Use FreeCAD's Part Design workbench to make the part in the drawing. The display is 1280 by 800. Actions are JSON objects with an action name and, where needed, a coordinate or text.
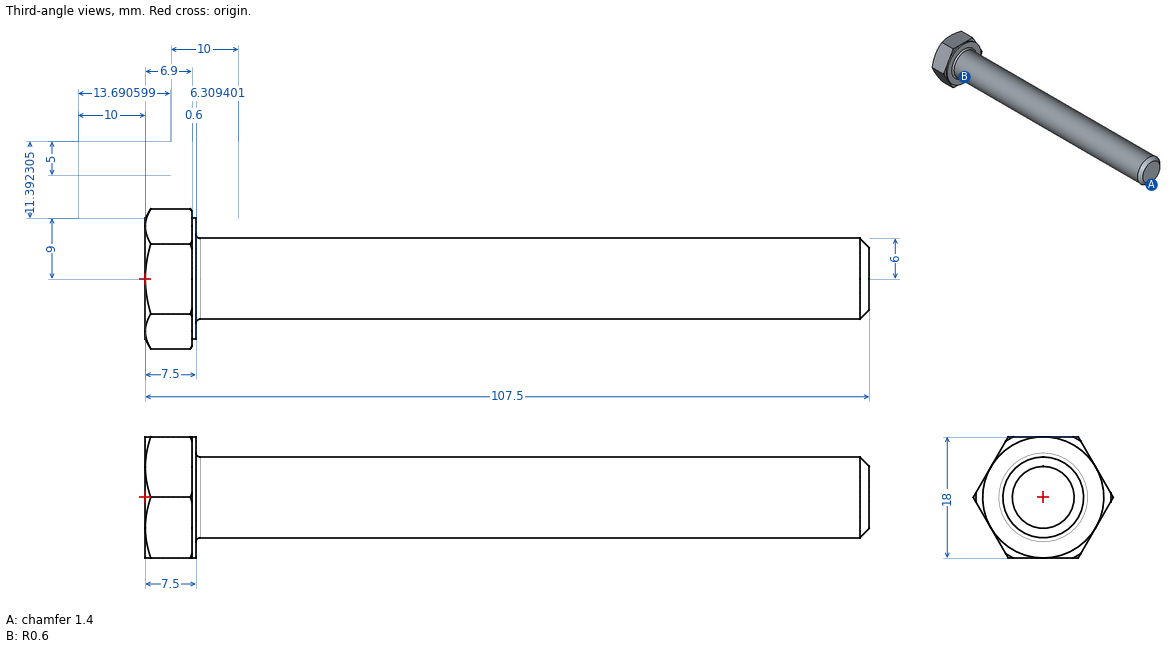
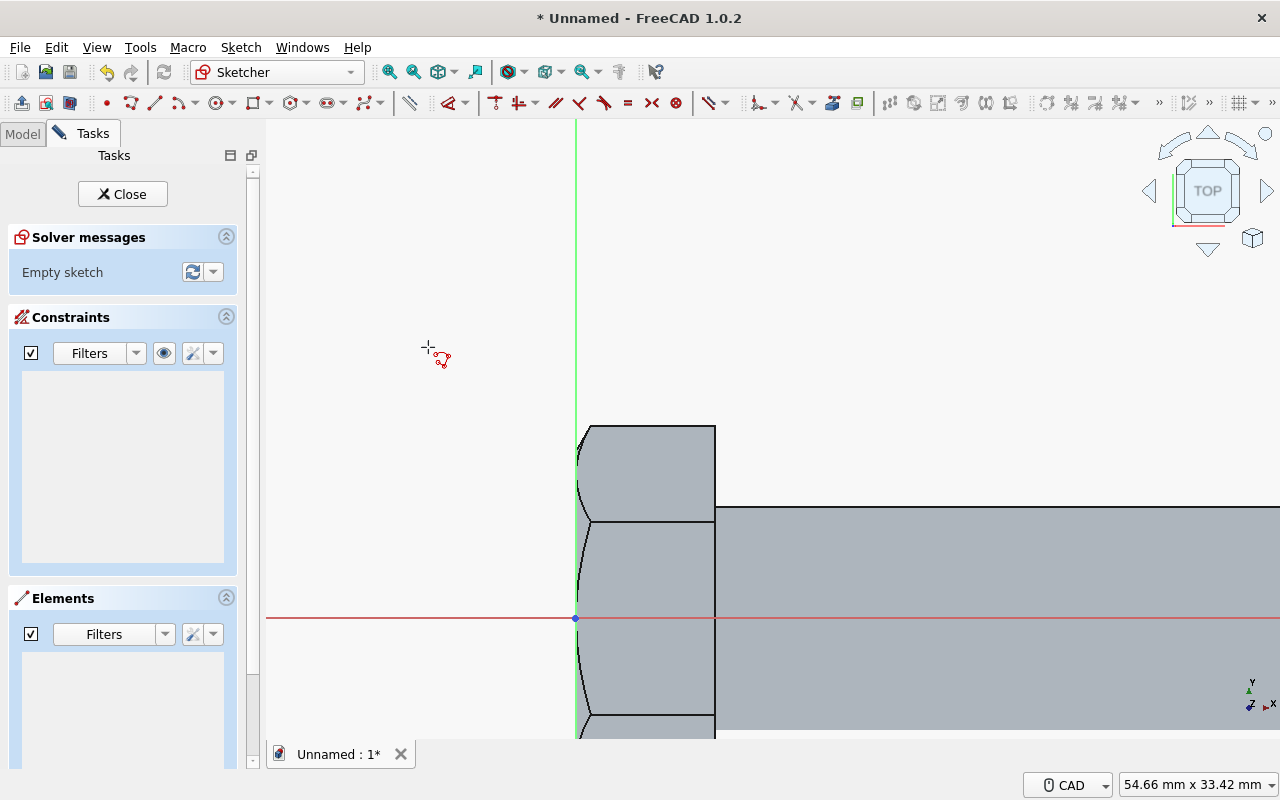
{"action": "left_click", "coordinate": [715, 451]}
{"action": "left_click", "coordinate": [832, 451]}
{"action": "left_click", "coordinate": [832, 240]}
{"action": "left_click", "coordinate": [647, 240]}
{"action": "left_click", "coordinate": [647, 333]}
{"action": "left_click", "coordinate": [715, 452]}
{"action": "key", "text": "Escape"}
{"action": "key", "text": "Escape"}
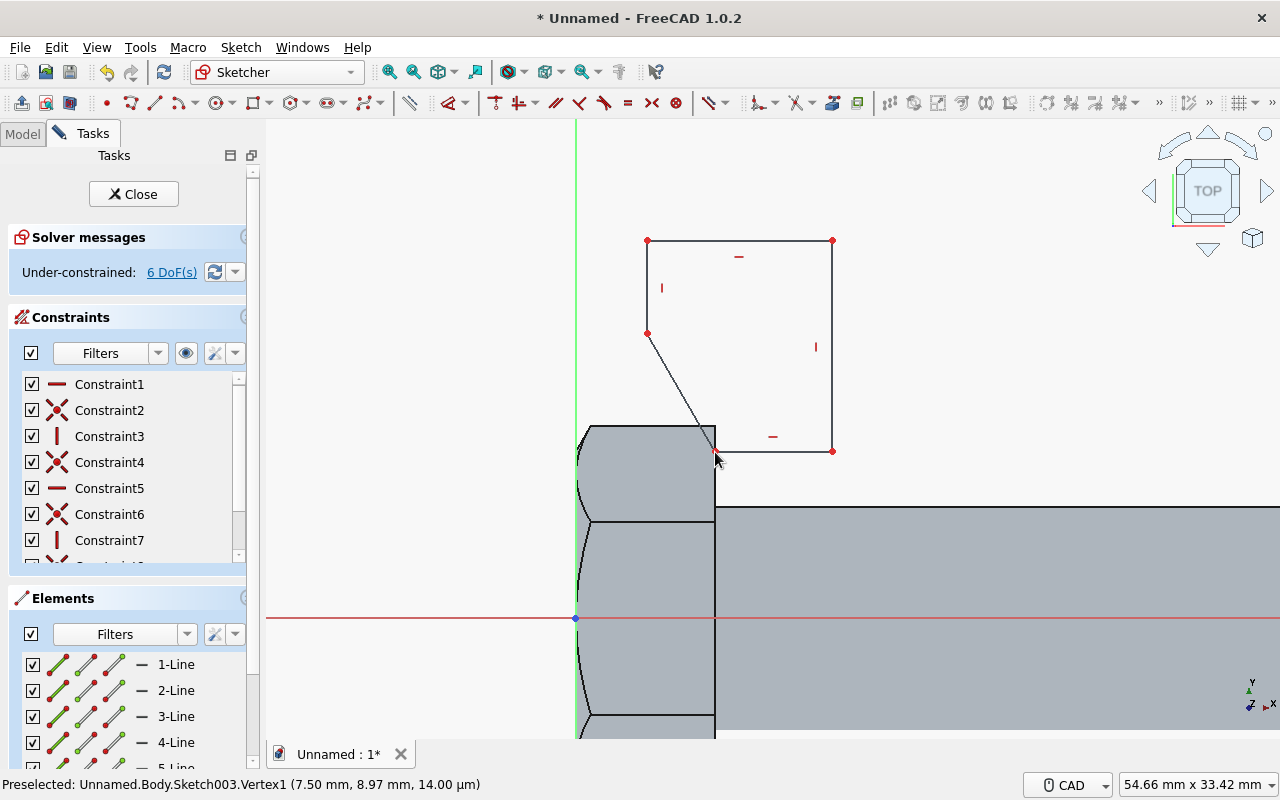
{"action": "key", "text": "d"}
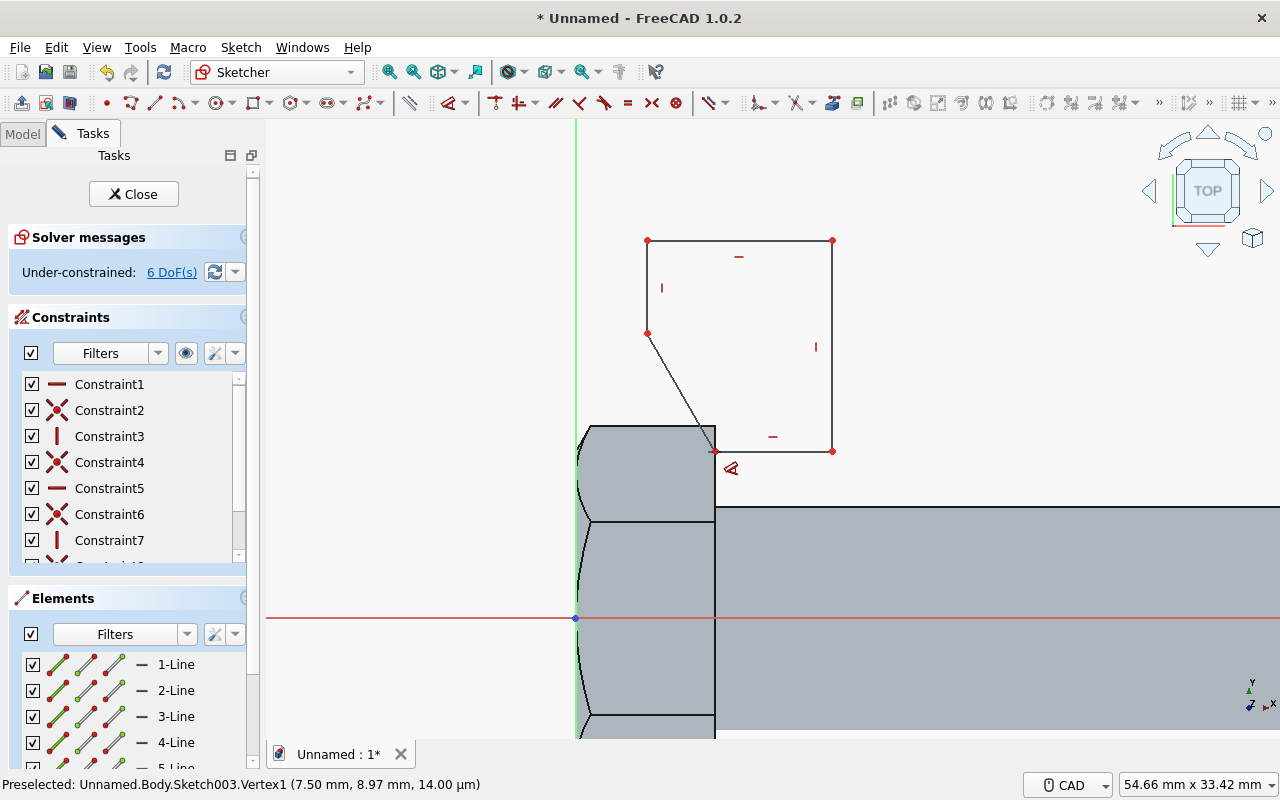
{"action": "left_click", "coordinate": [647, 269]}
{"action": "left_click", "coordinate": [613, 288]}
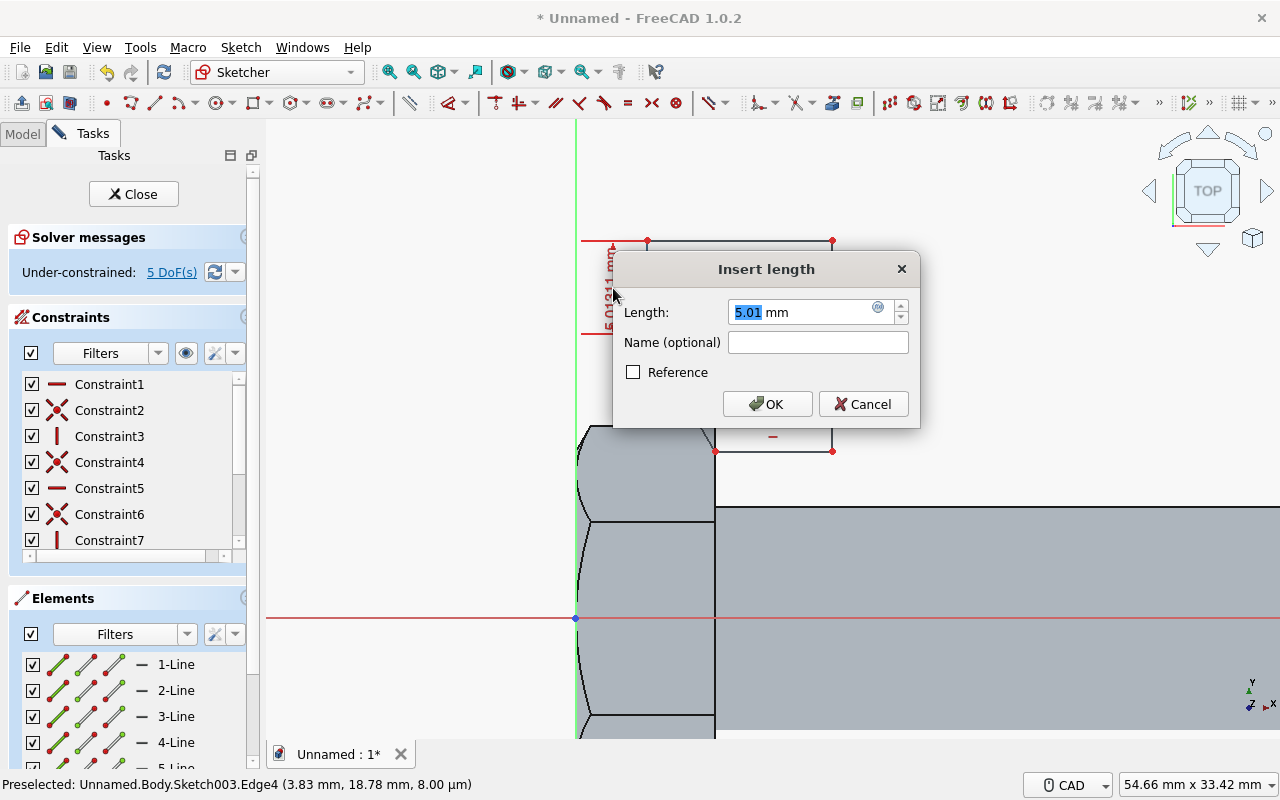
{"action": "type", "text": "5"}
{"action": "key", "text": "Return"}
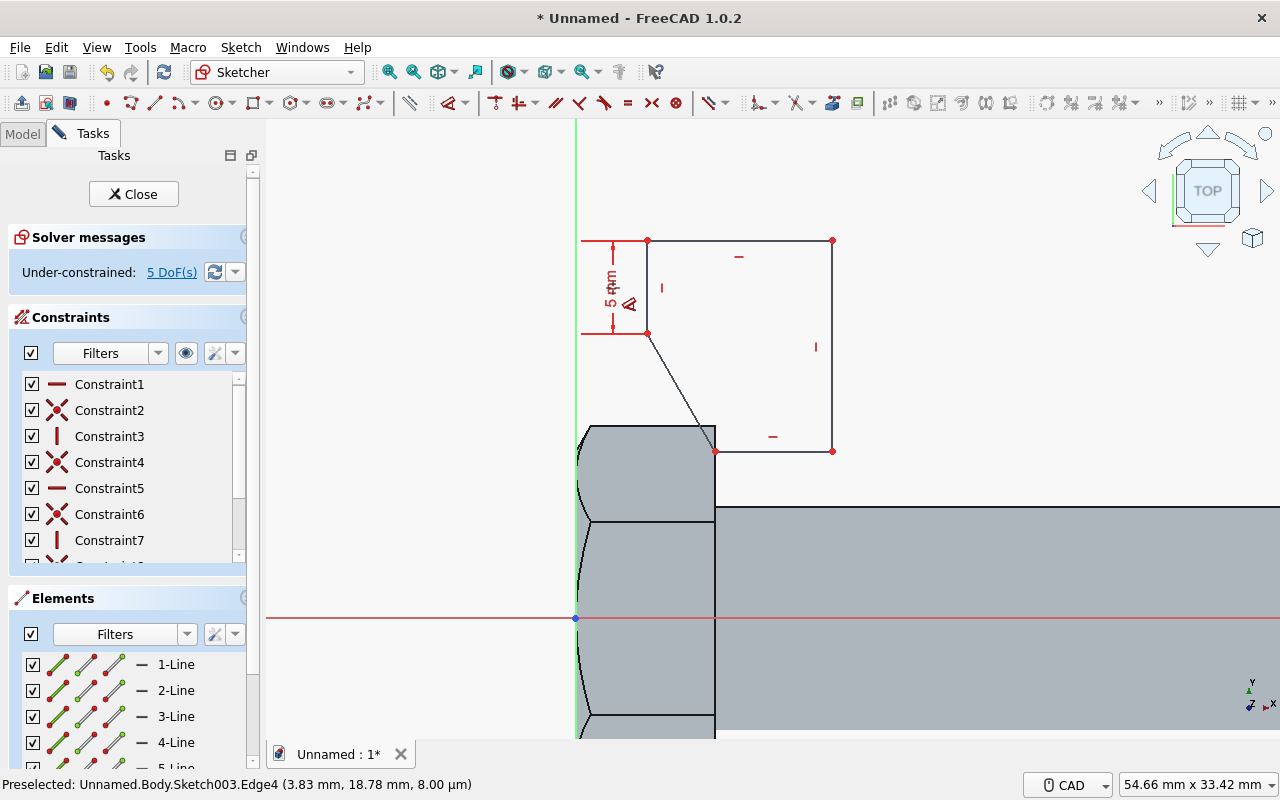
{"action": "left_click", "coordinate": [776, 241]}
{"action": "left_click", "coordinate": [739, 207]}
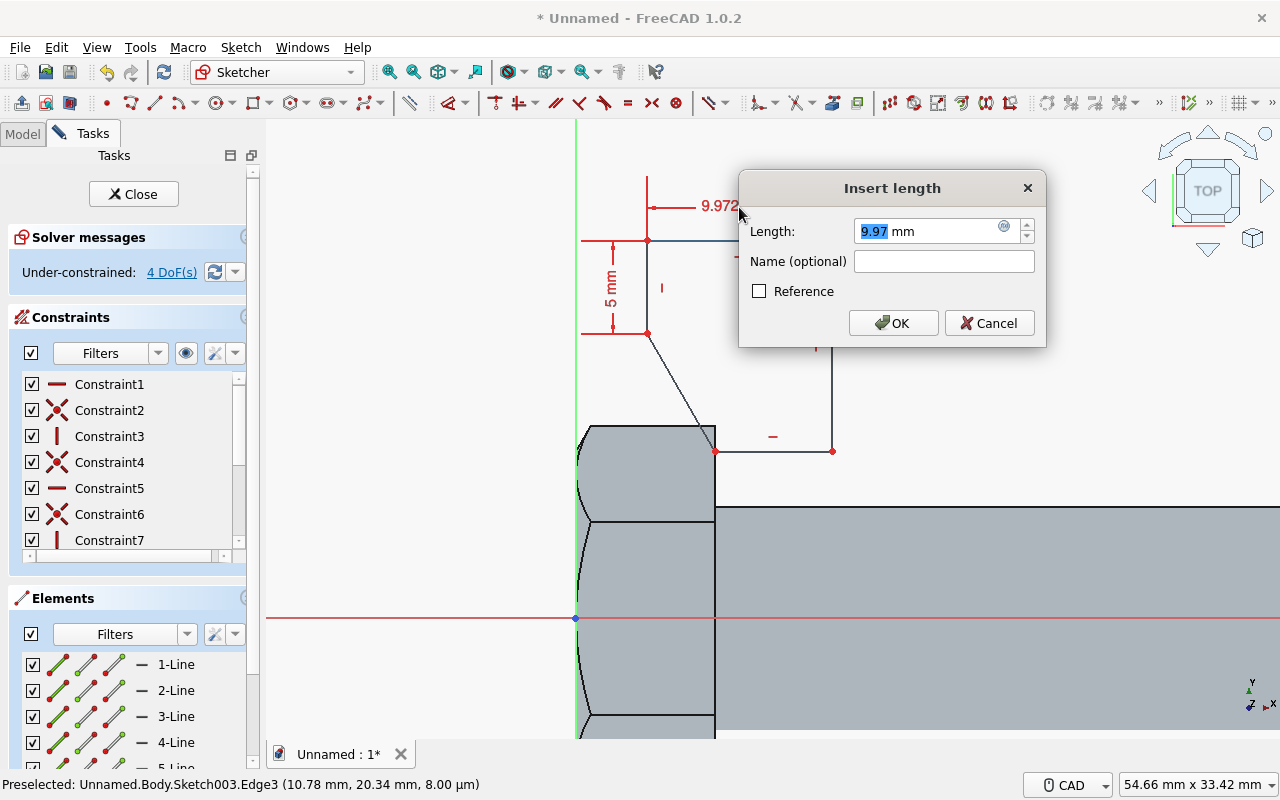
{"action": "type", "text": "10"}
{"action": "key", "text": "Return"}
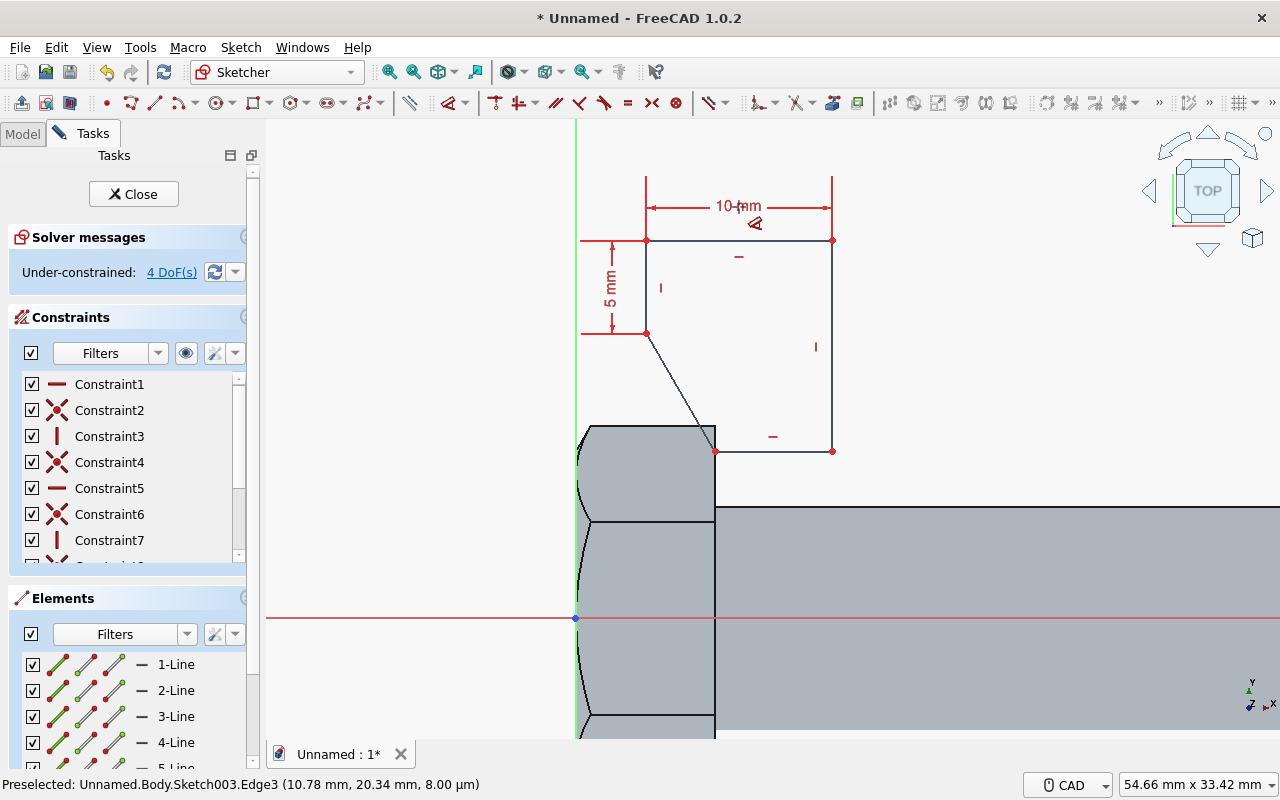
{"action": "left_click", "coordinate": [715, 452]}
{"action": "left_click", "coordinate": [542, 535]}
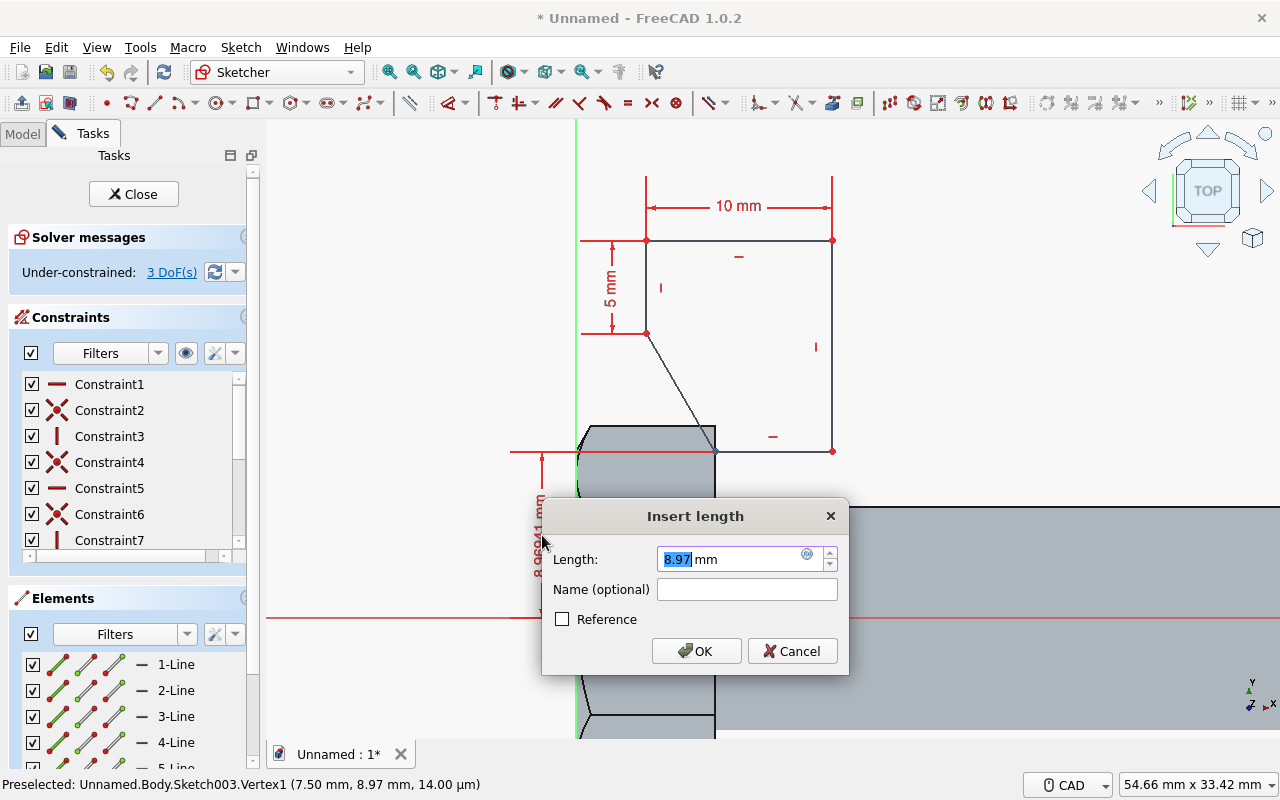
{"action": "type", "text": "9"}
{"action": "key", "text": "Return"}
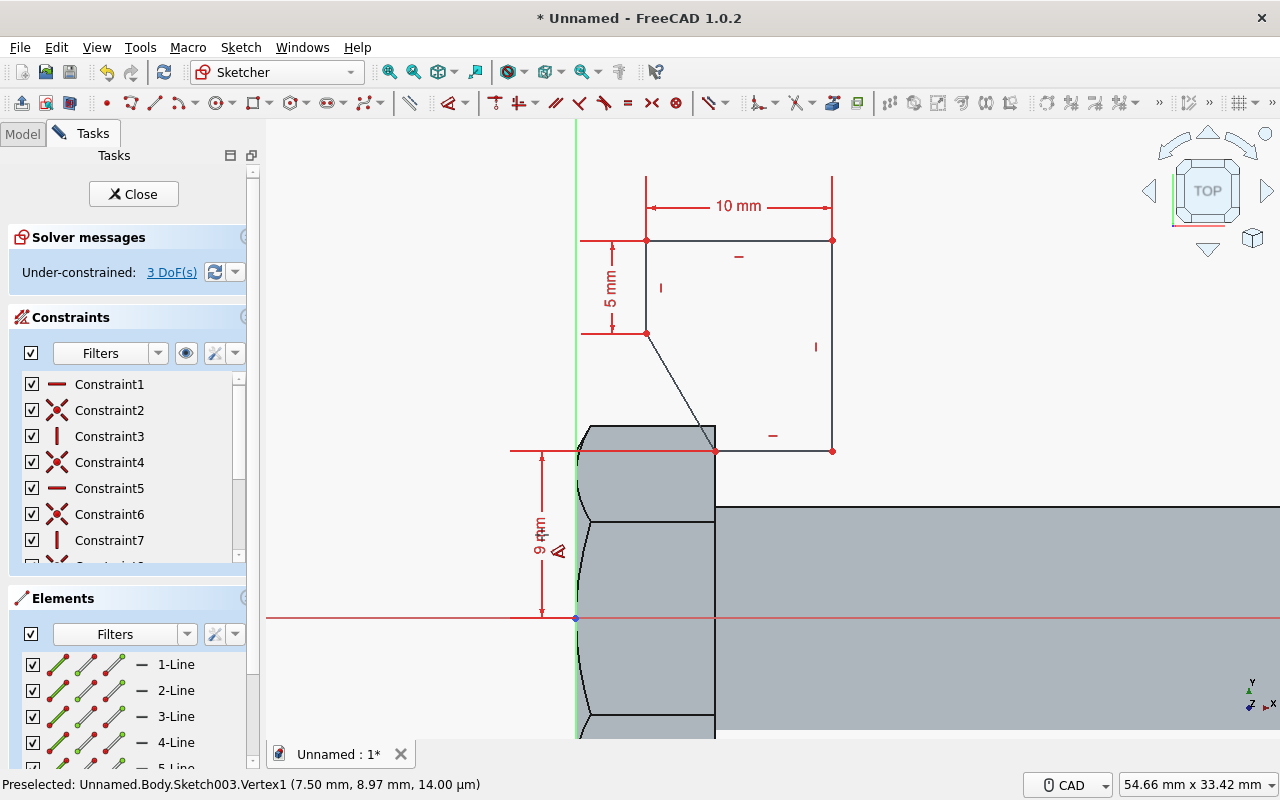
{"action": "left_click", "coordinate": [715, 451]}
{"action": "left_click", "coordinate": [645, 652]}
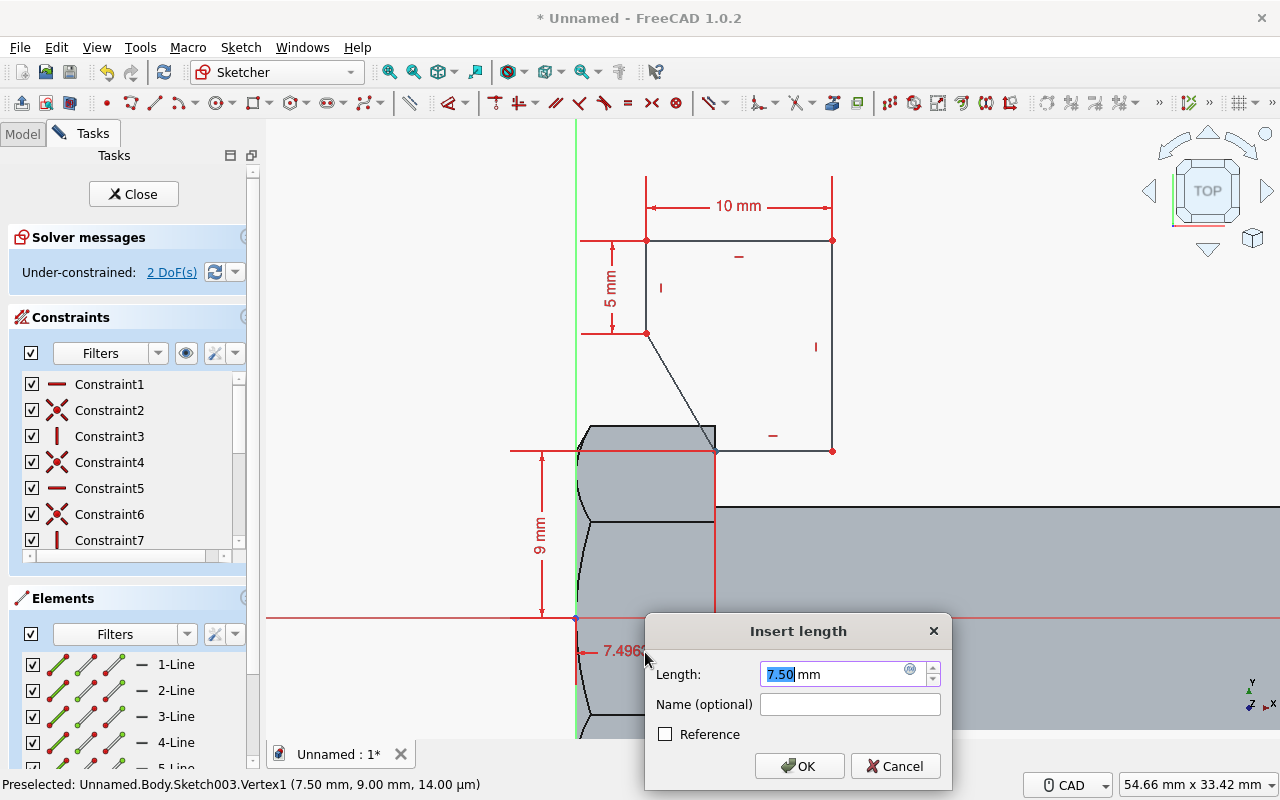
{"action": "type", "text": "7.5"}
{"action": "key", "text": "Return"}